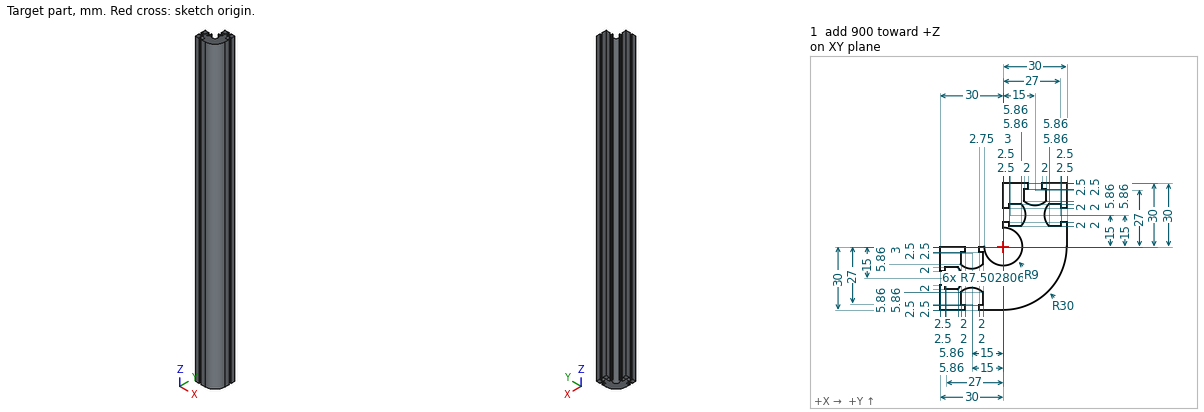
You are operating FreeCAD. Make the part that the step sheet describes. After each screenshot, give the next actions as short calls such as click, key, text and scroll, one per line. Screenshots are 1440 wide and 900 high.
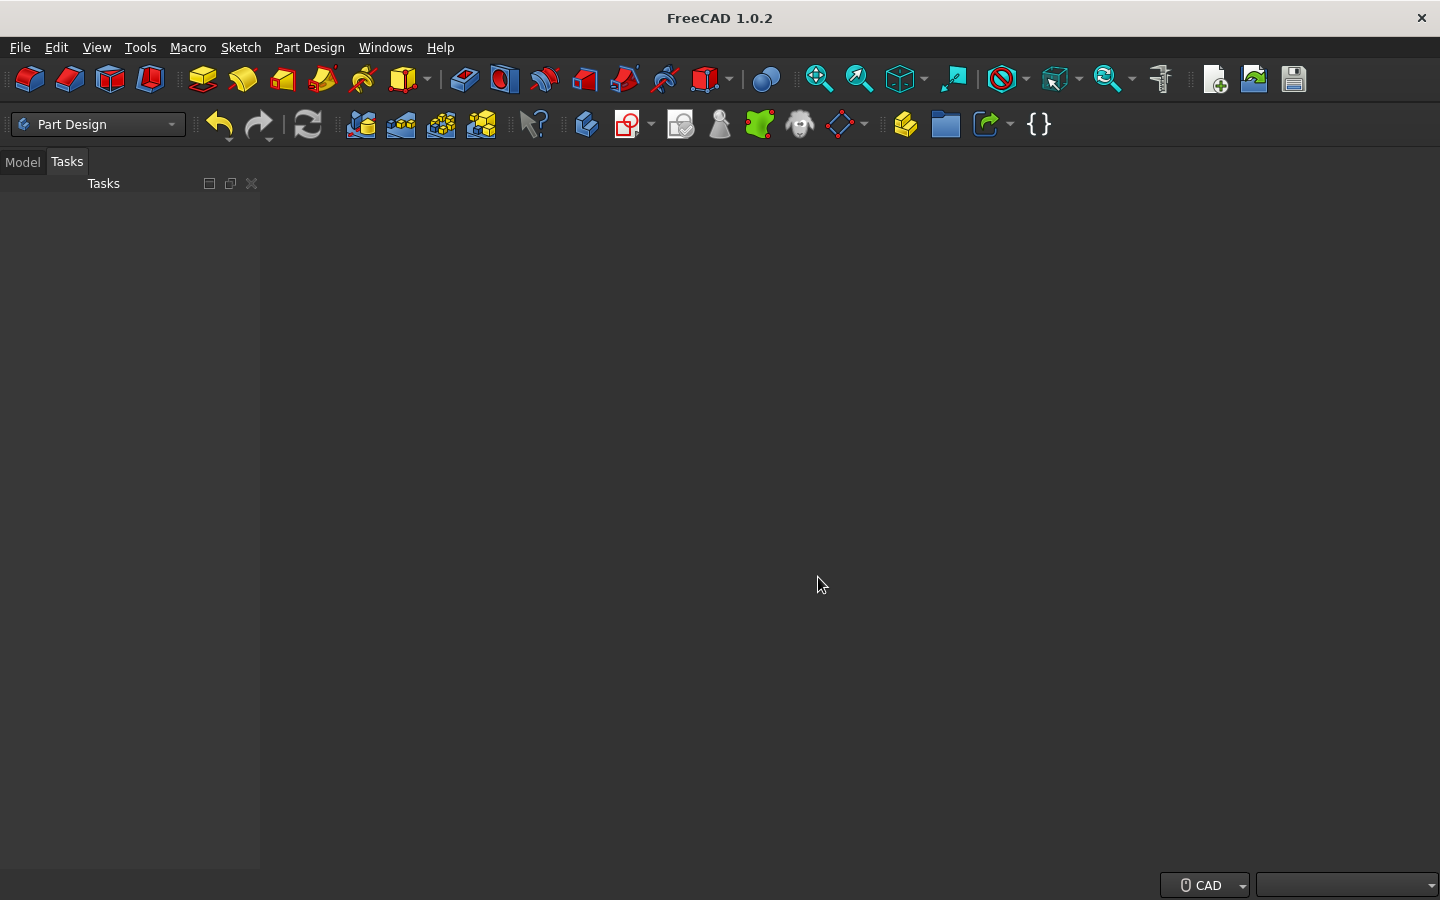
click(1214, 80)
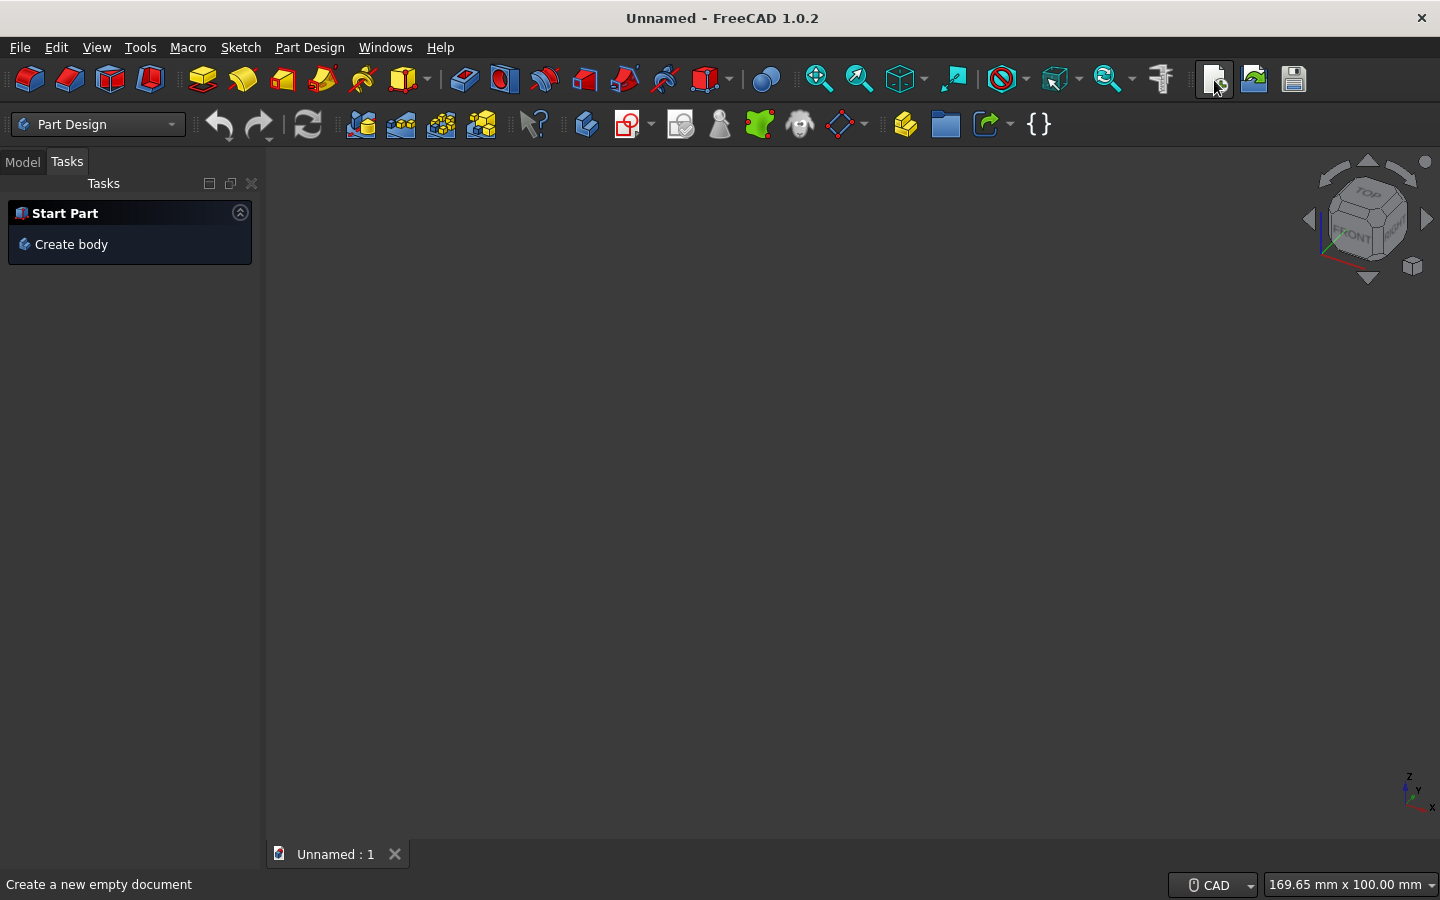
click(628, 124)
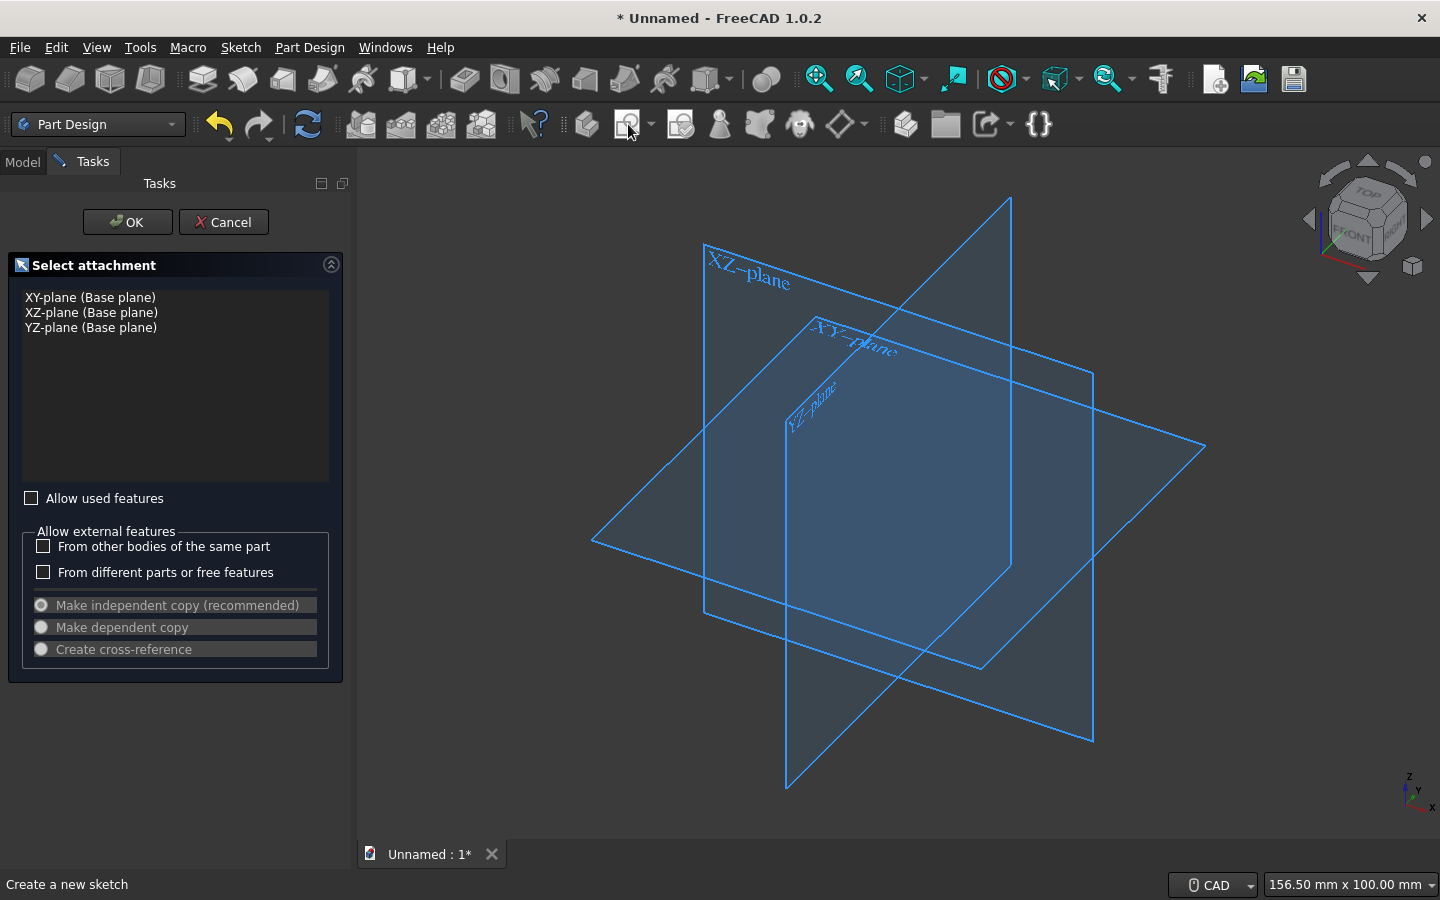
click(82, 298)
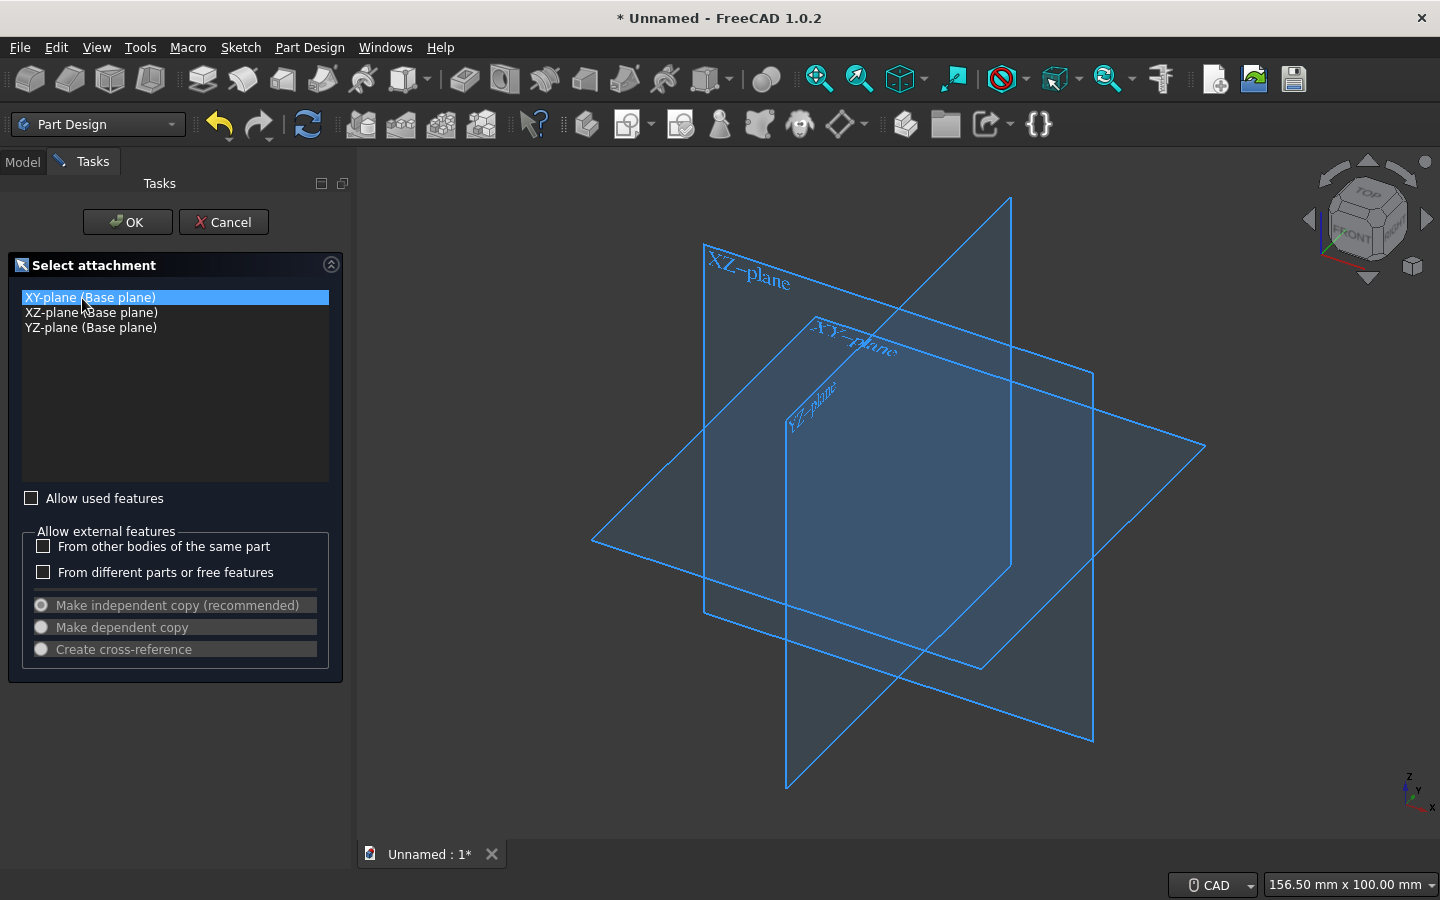
click(128, 222)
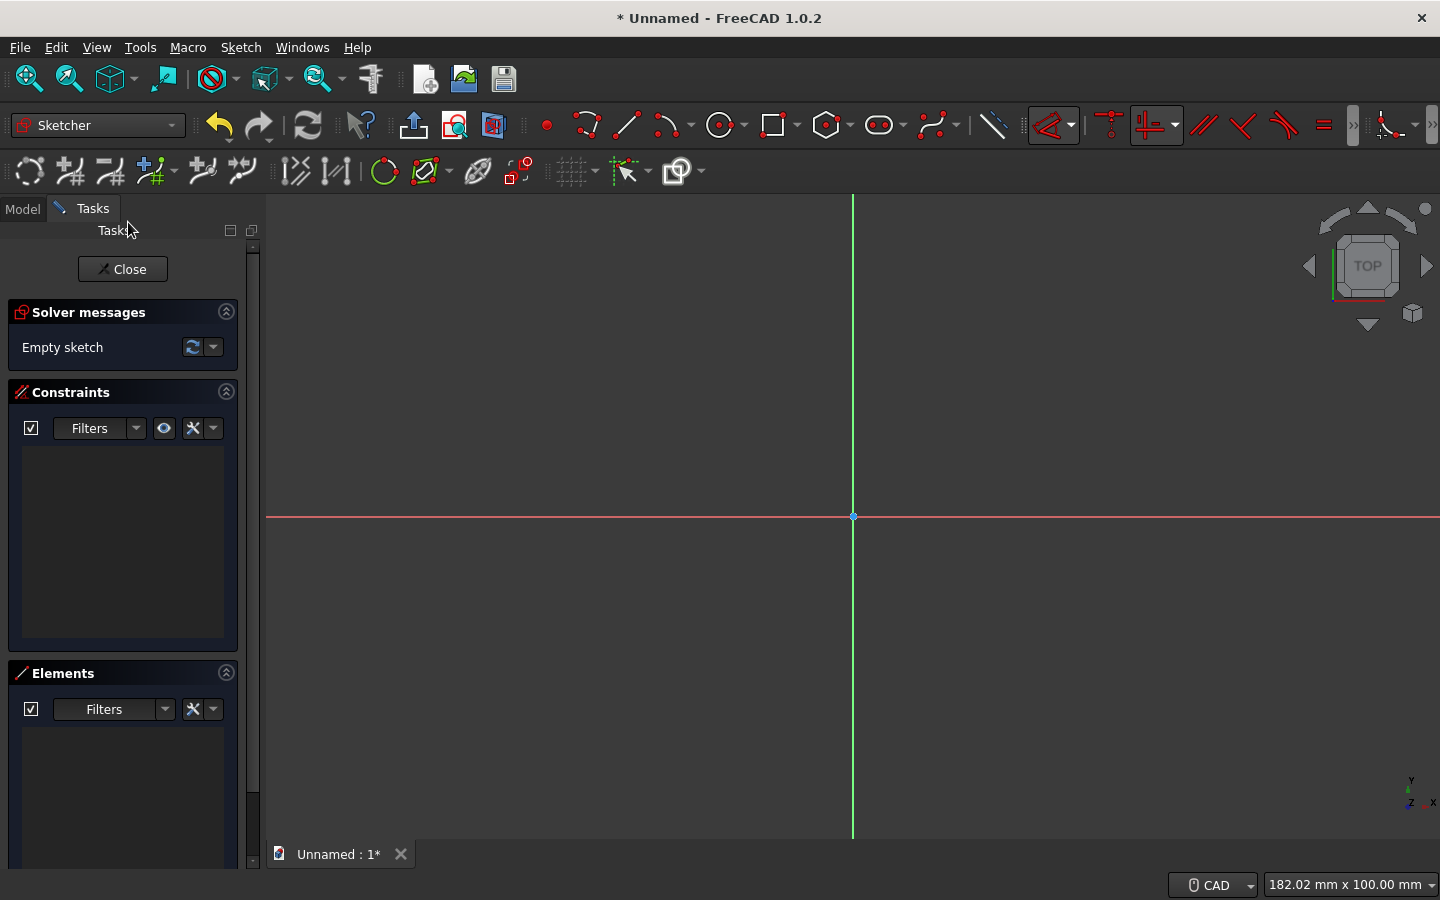
click(588, 126)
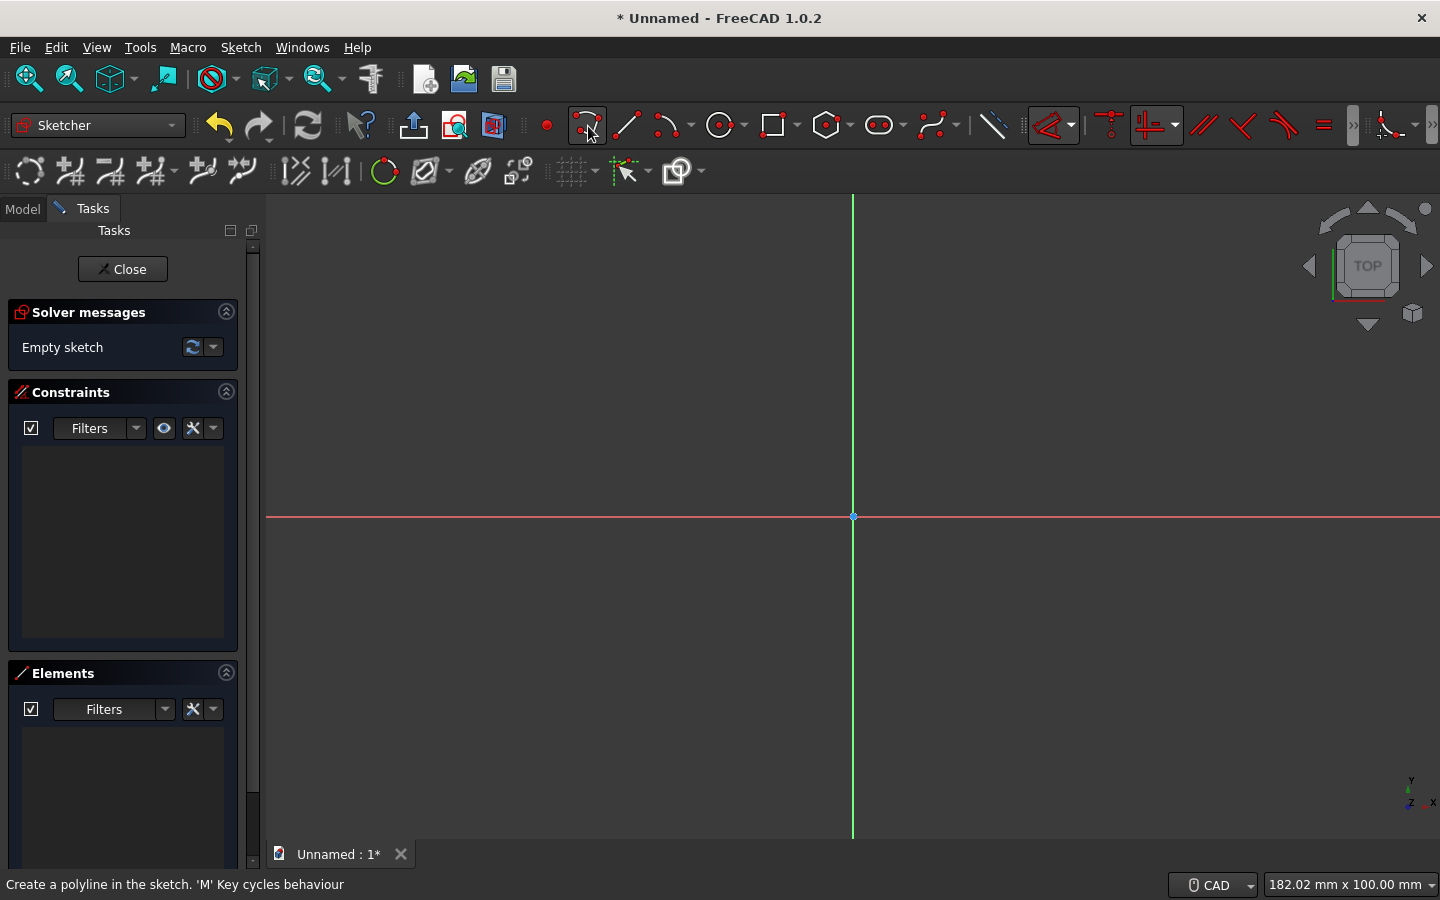
click(795, 516)
click(777, 508)
click(777, 533)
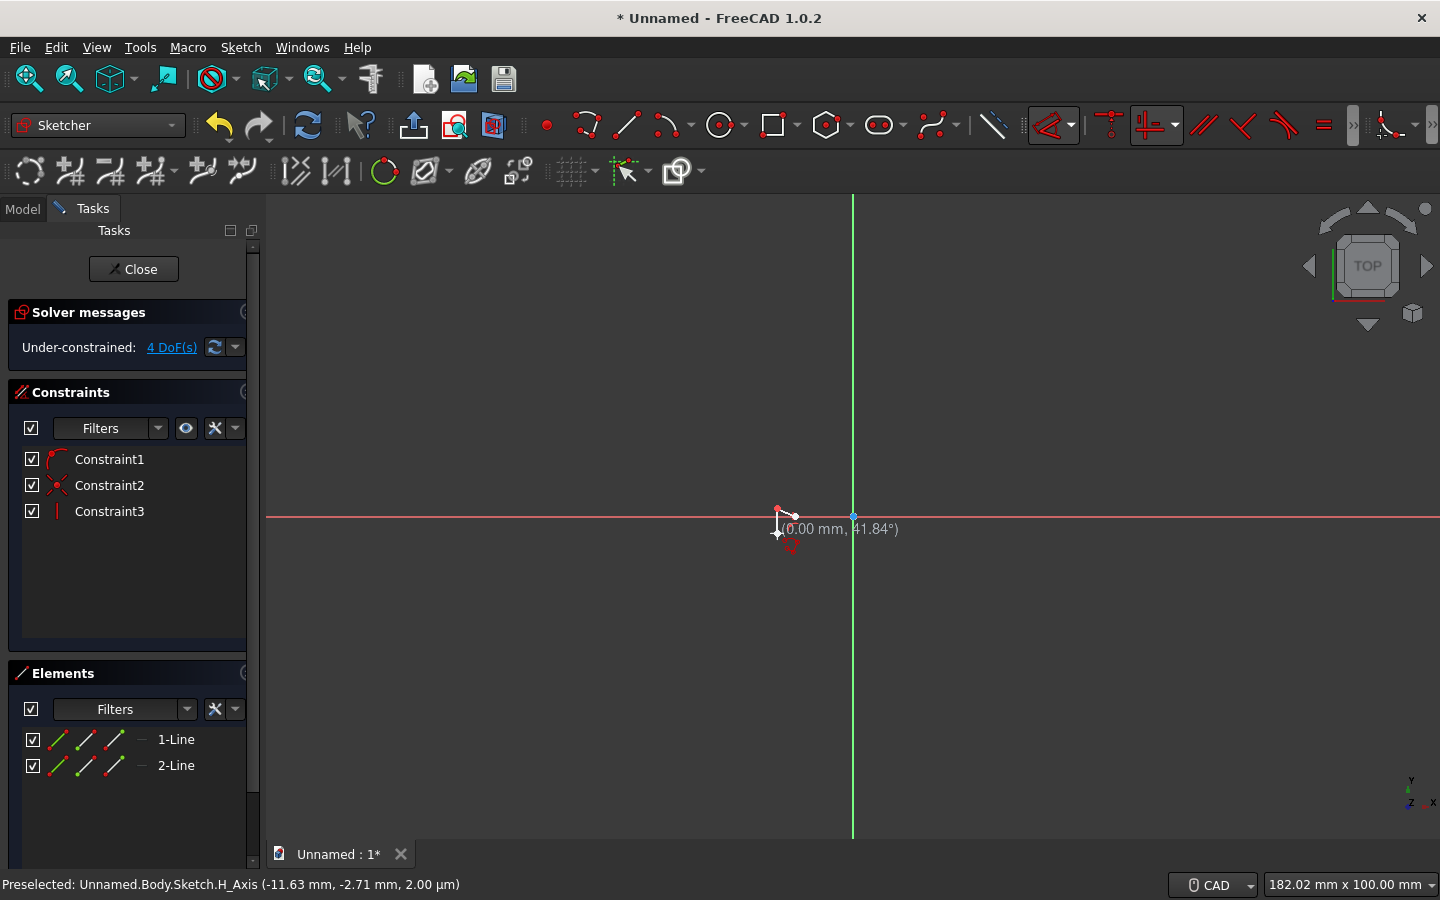
scroll(790, 533, up, 2)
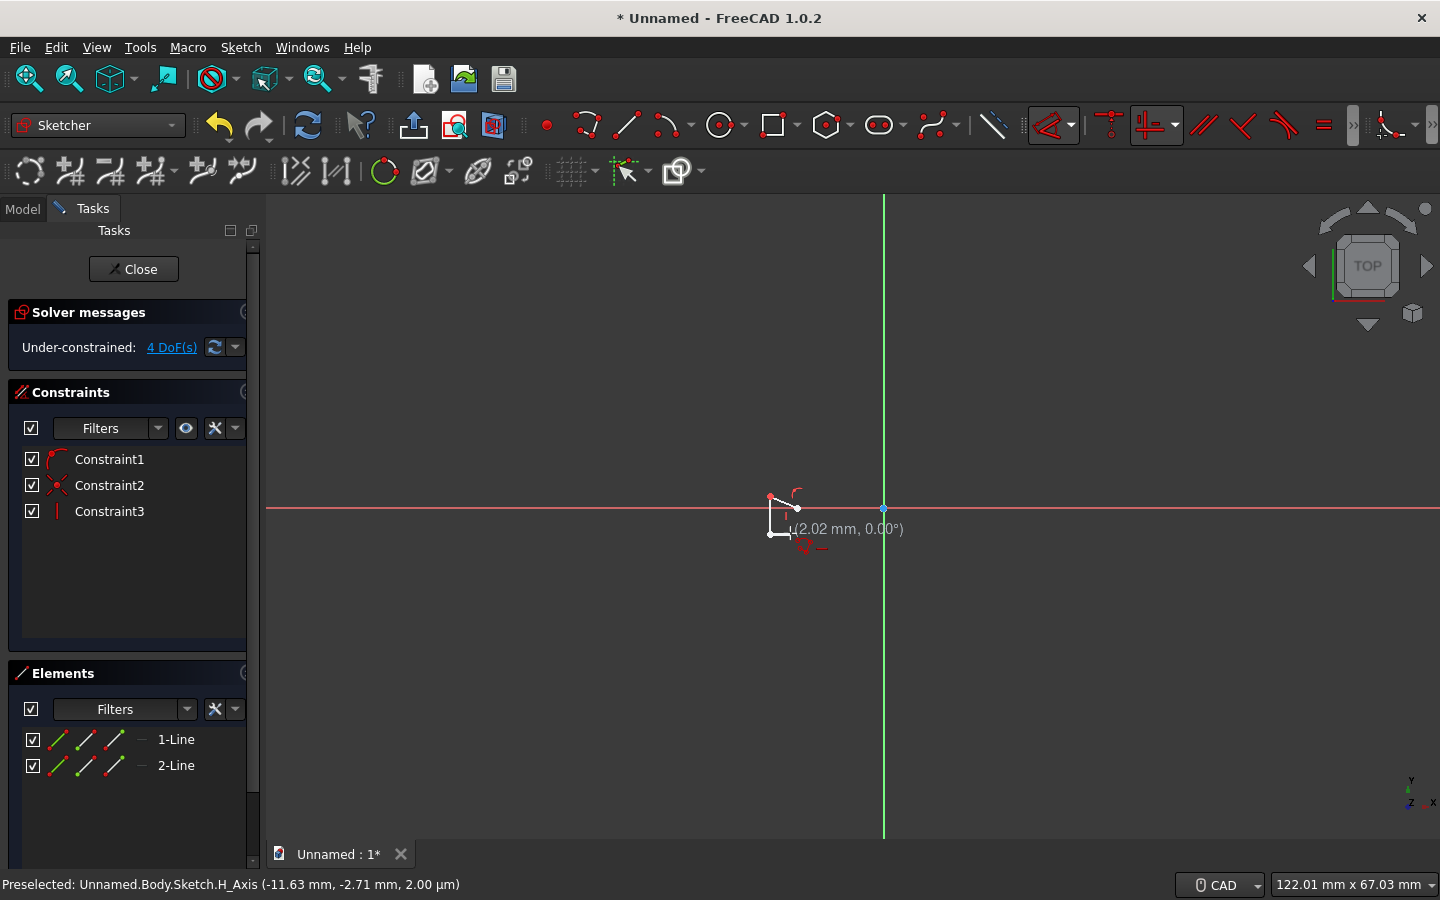
click(790, 533)
click(790, 589)
right_click(790, 589)